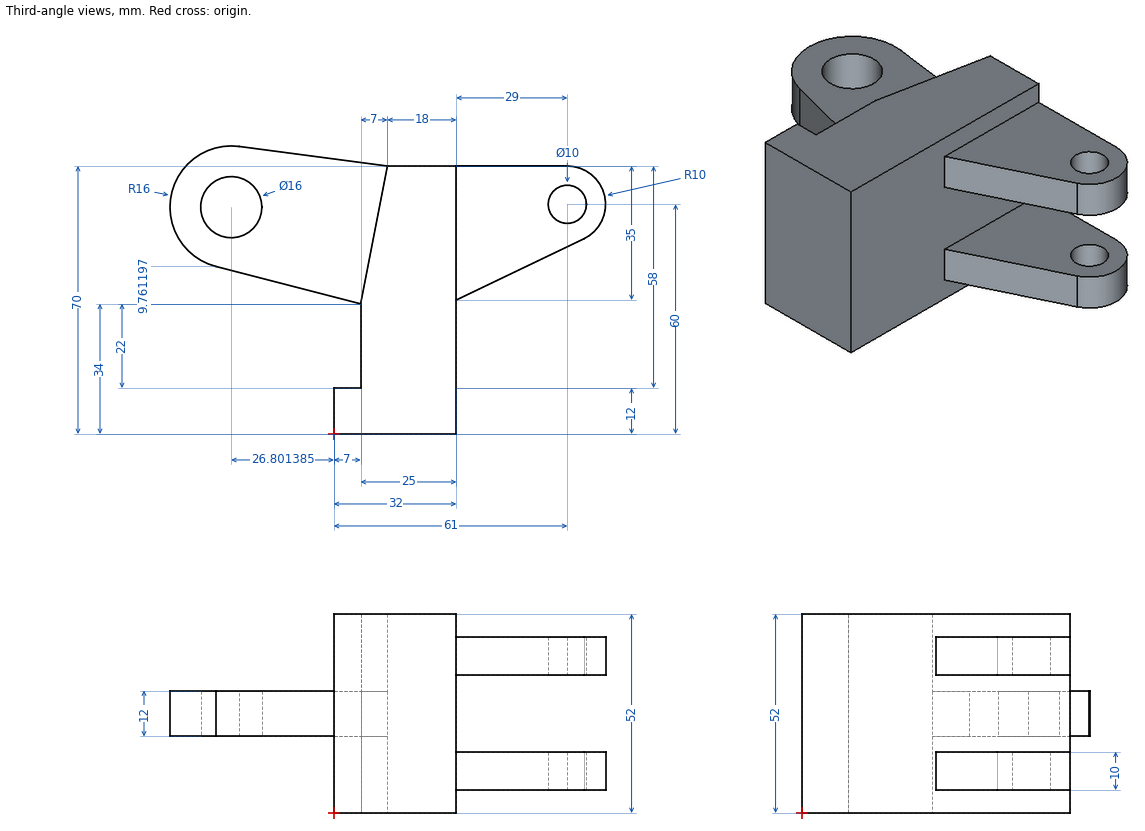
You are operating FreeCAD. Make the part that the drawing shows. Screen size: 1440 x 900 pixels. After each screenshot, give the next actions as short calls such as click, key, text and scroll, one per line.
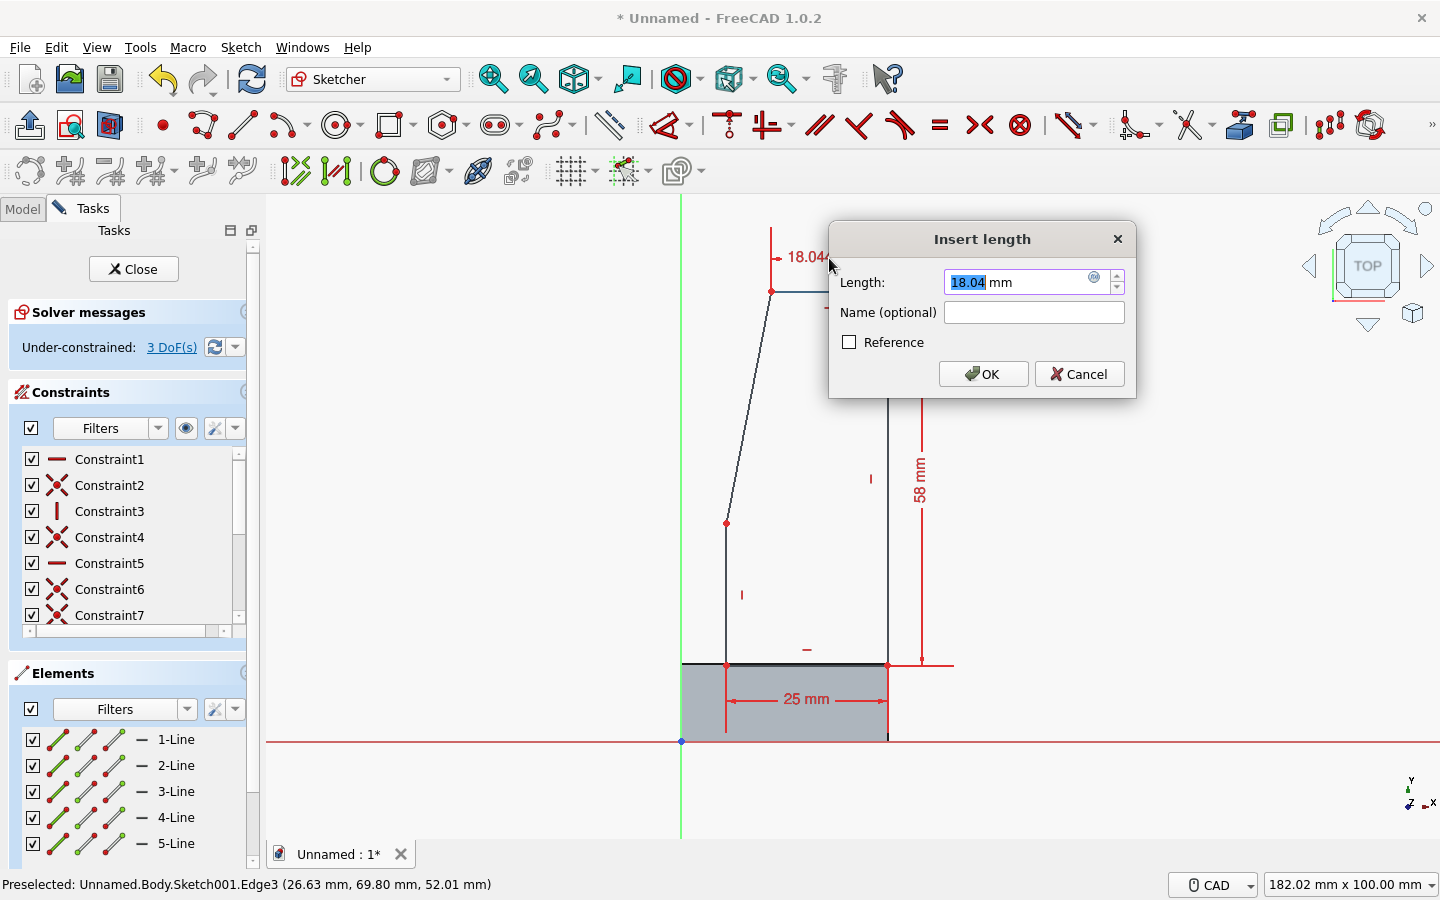
text(18)
key(Return)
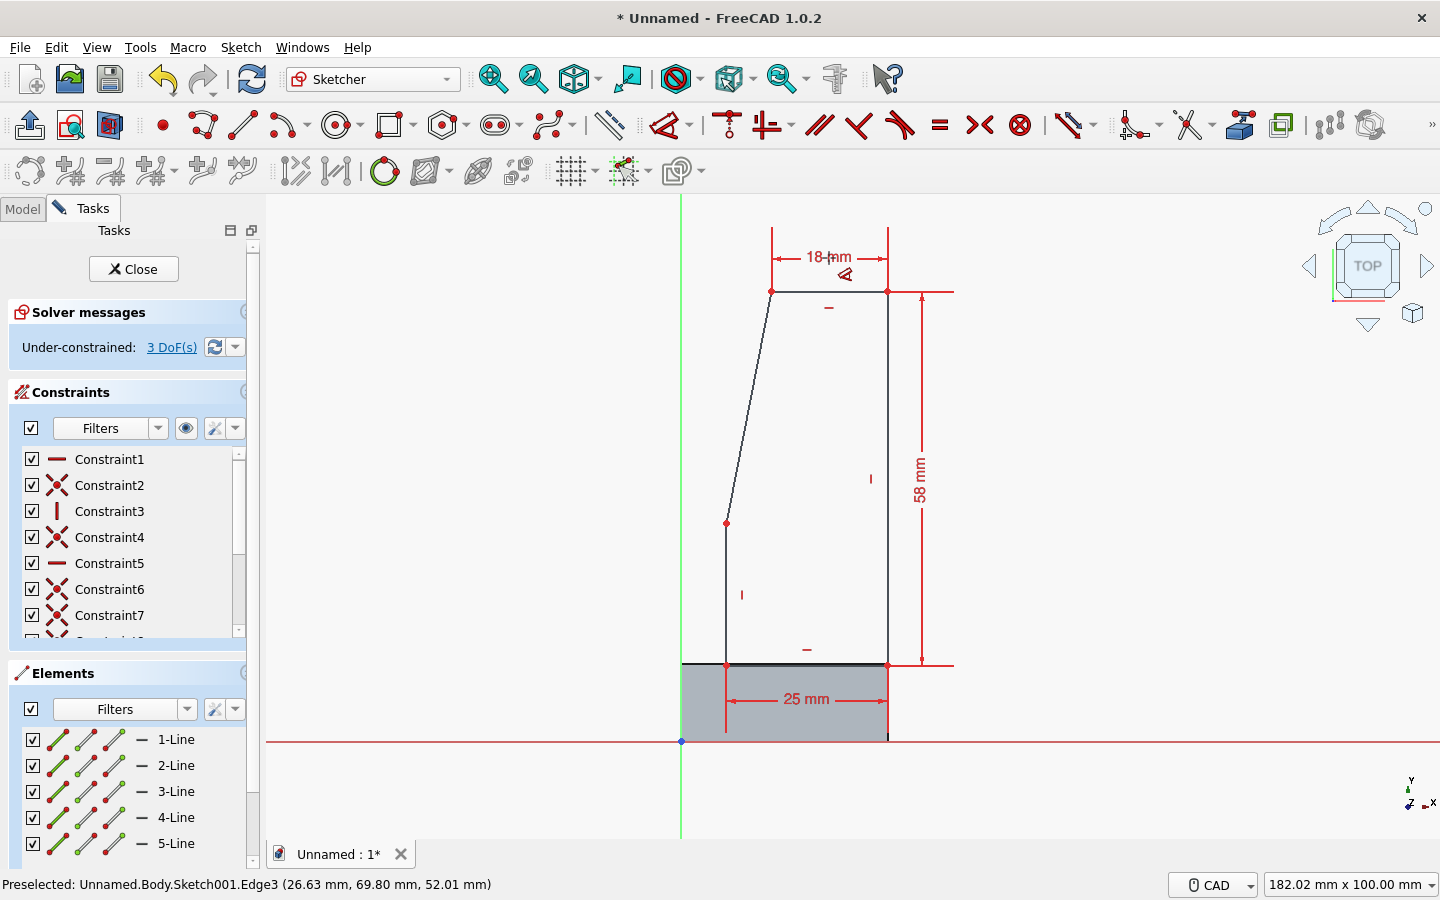
click(726, 567)
click(760, 595)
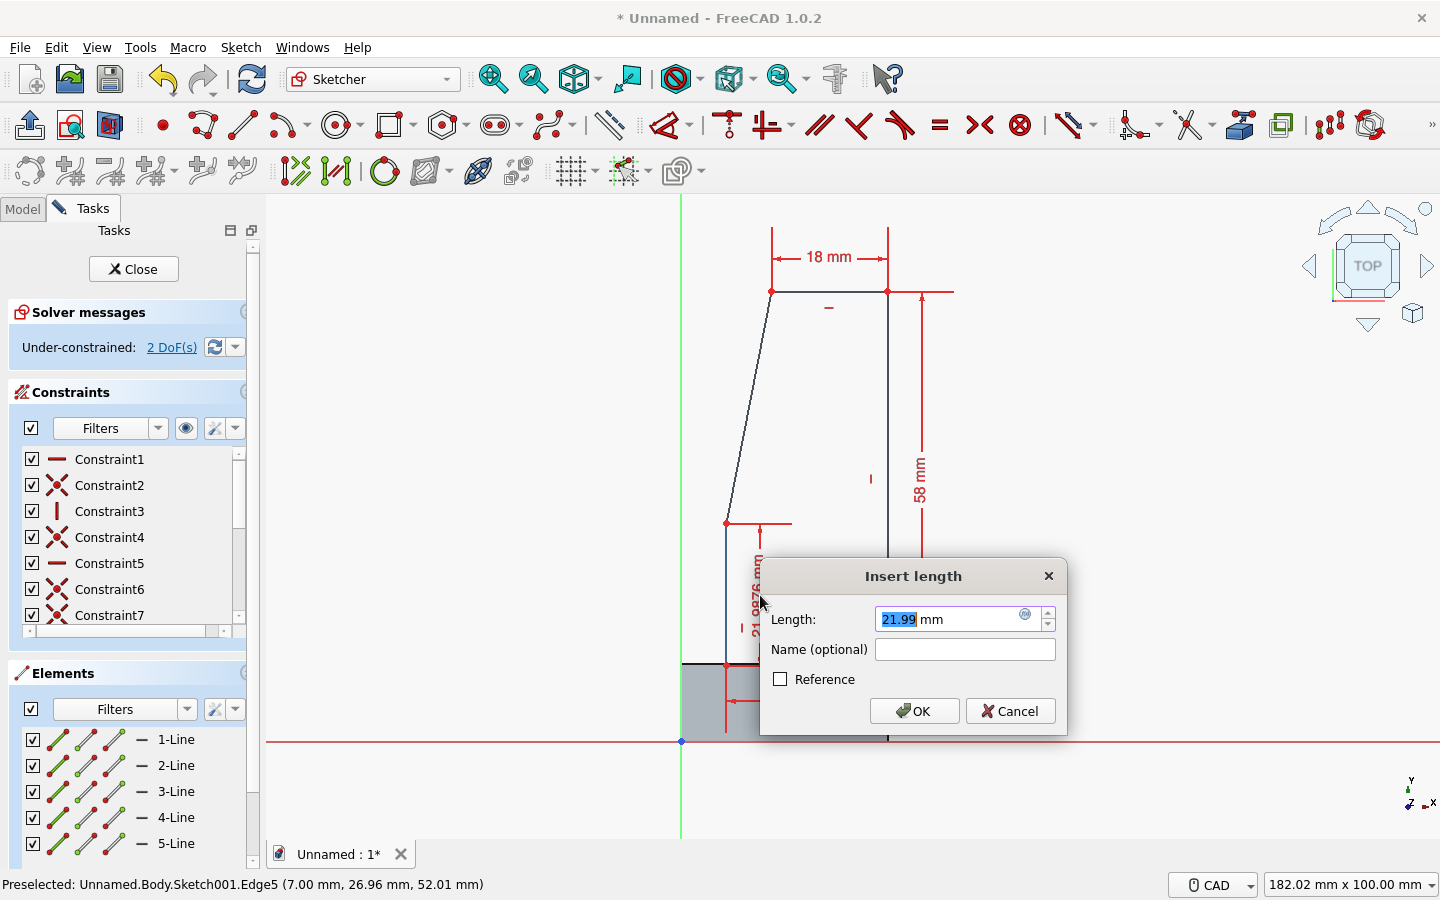
text(22)
key(Return)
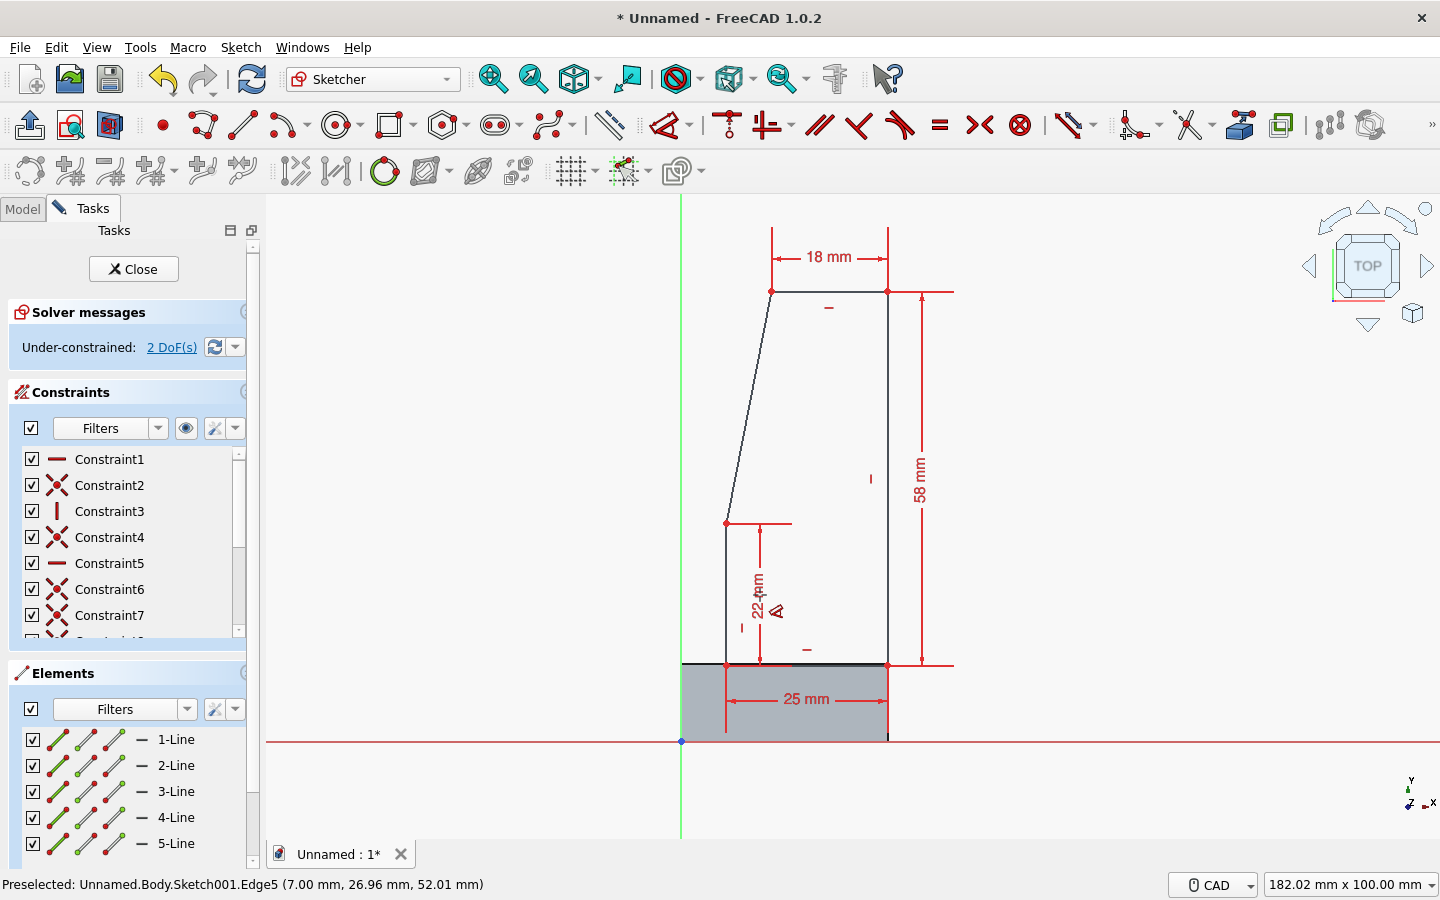
click(726, 666)
click(704, 776)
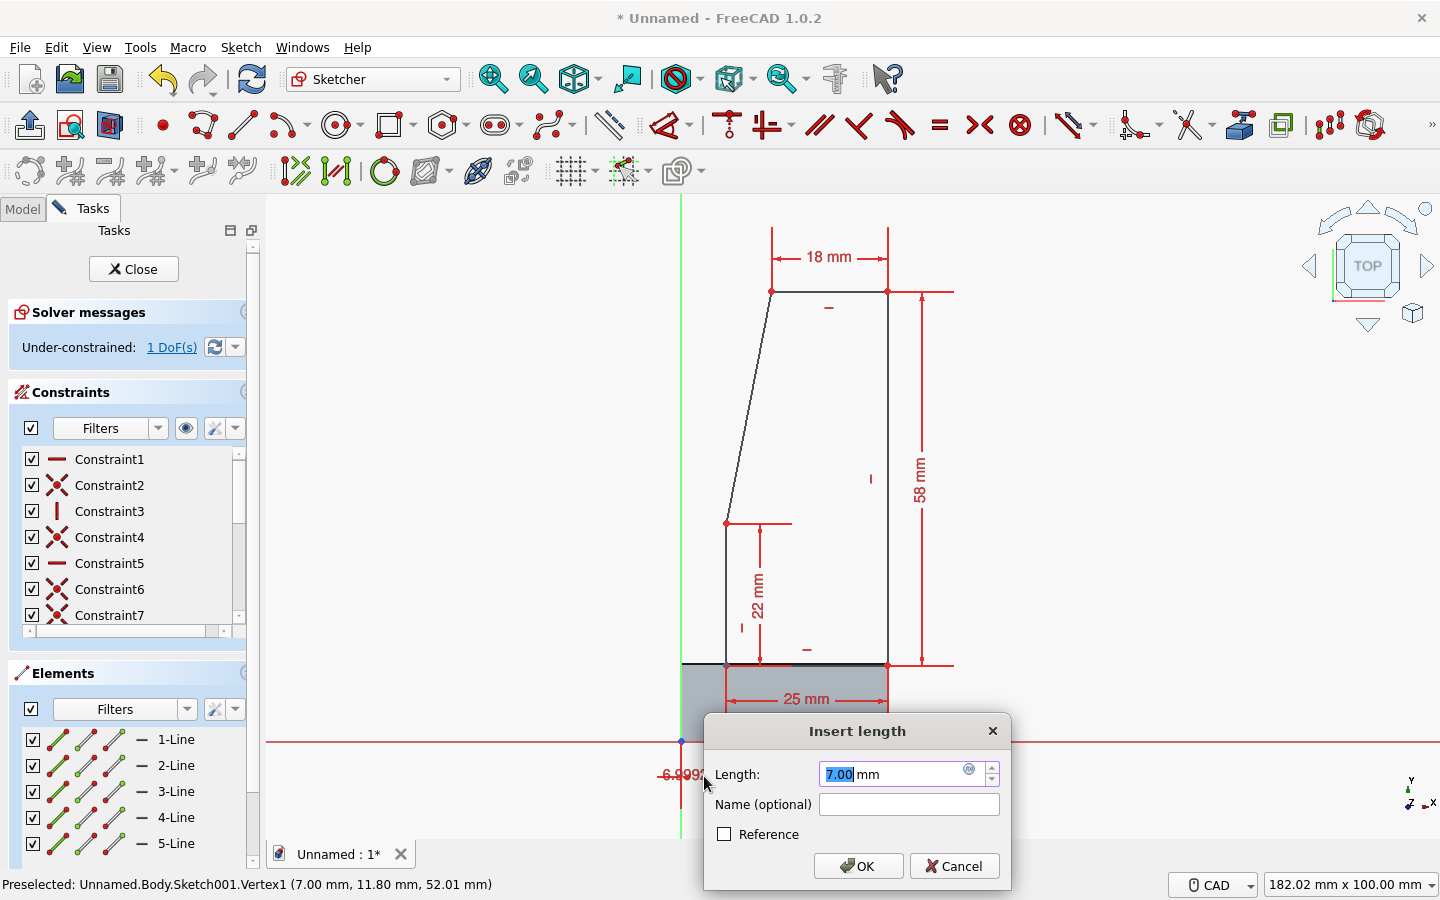
text(7)
key(Return)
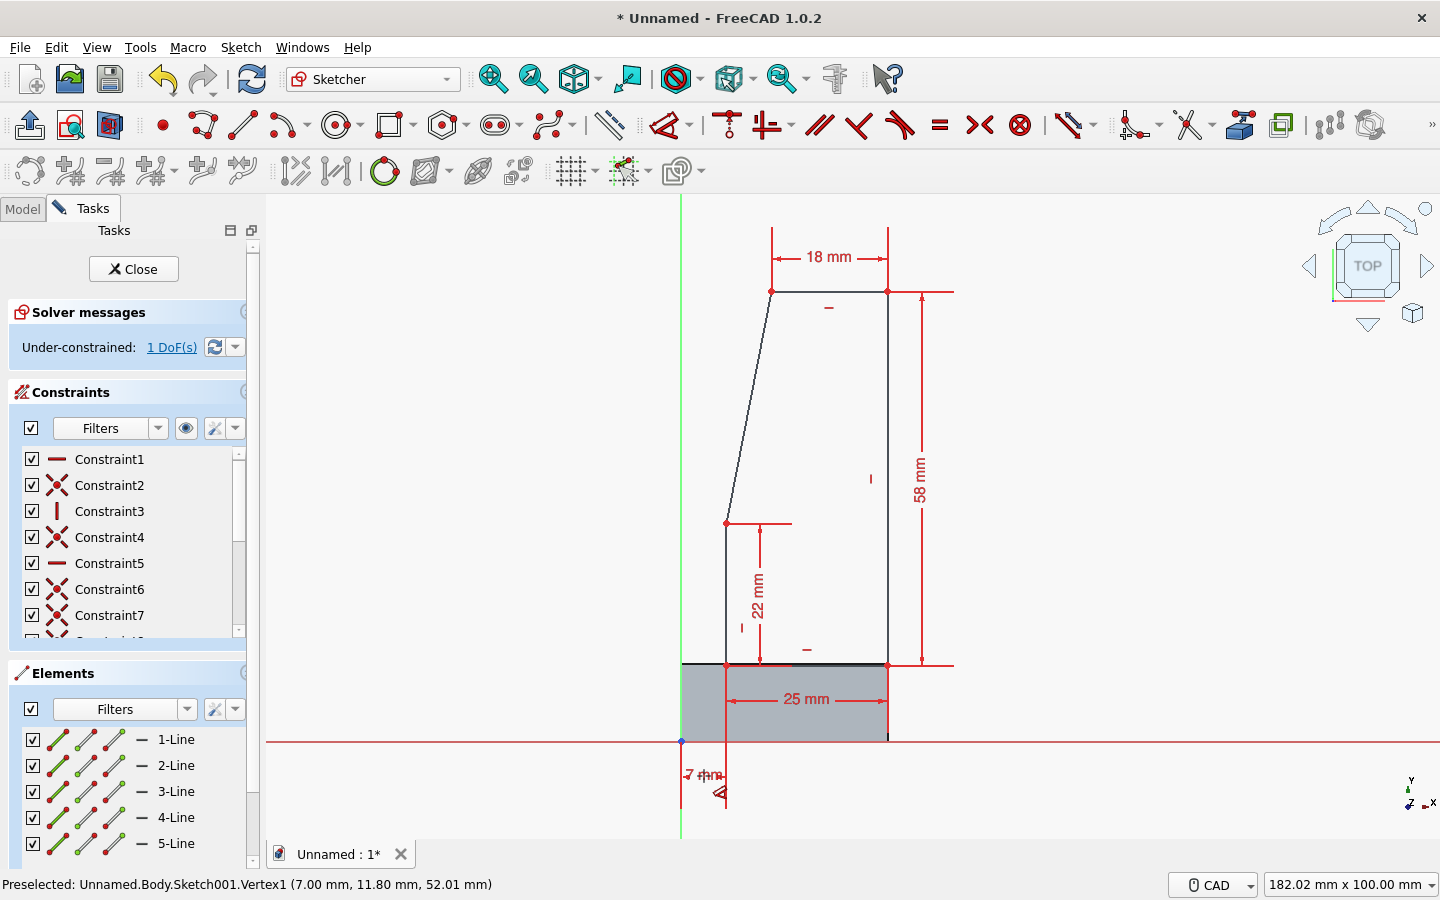
click(726, 666)
click(647, 704)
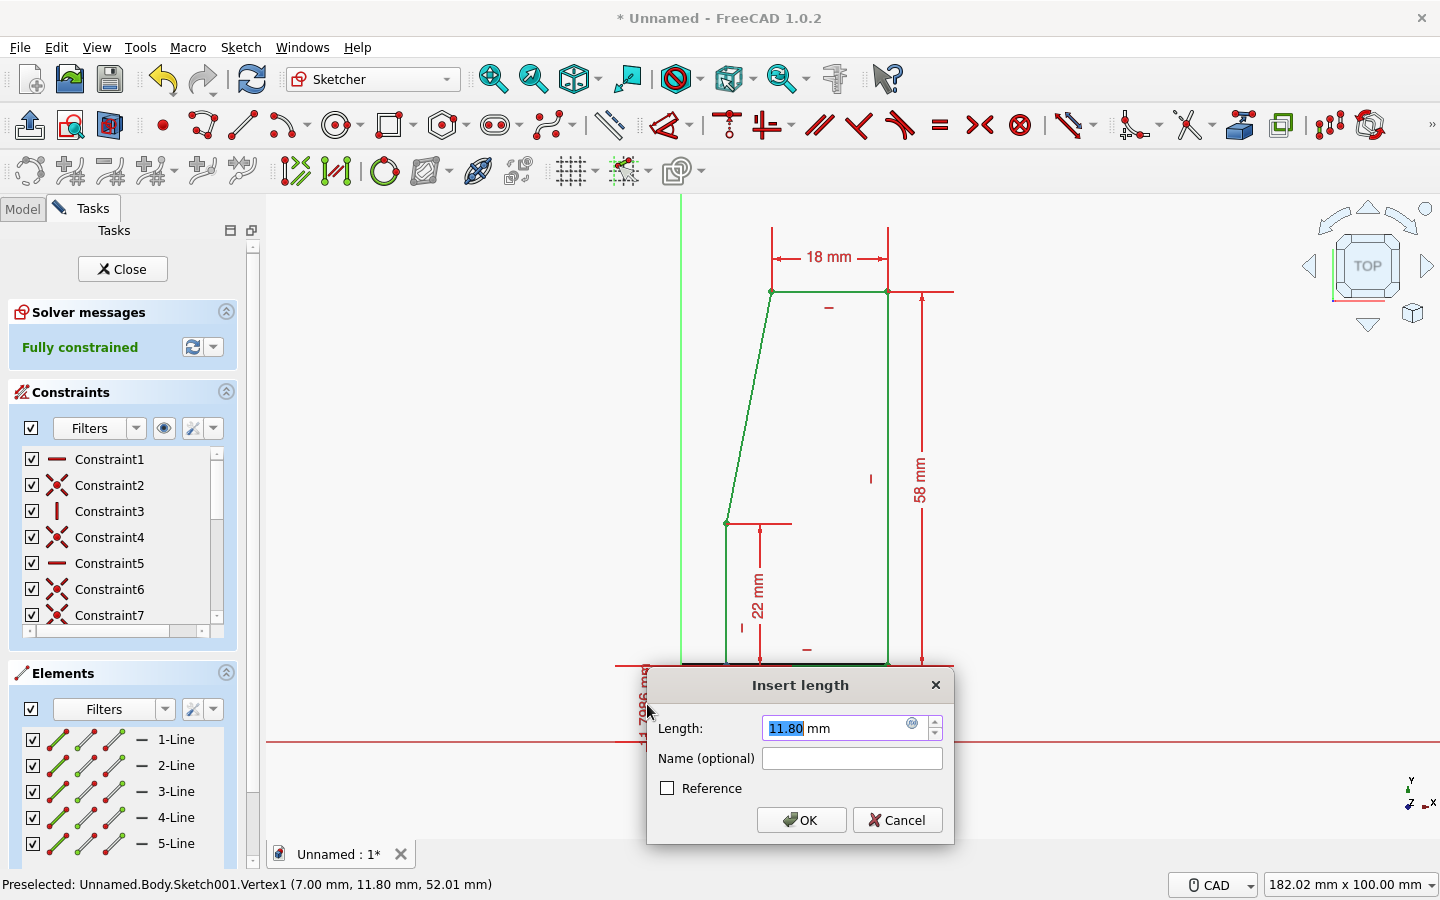
text(12)
key(Return)
key(Escape)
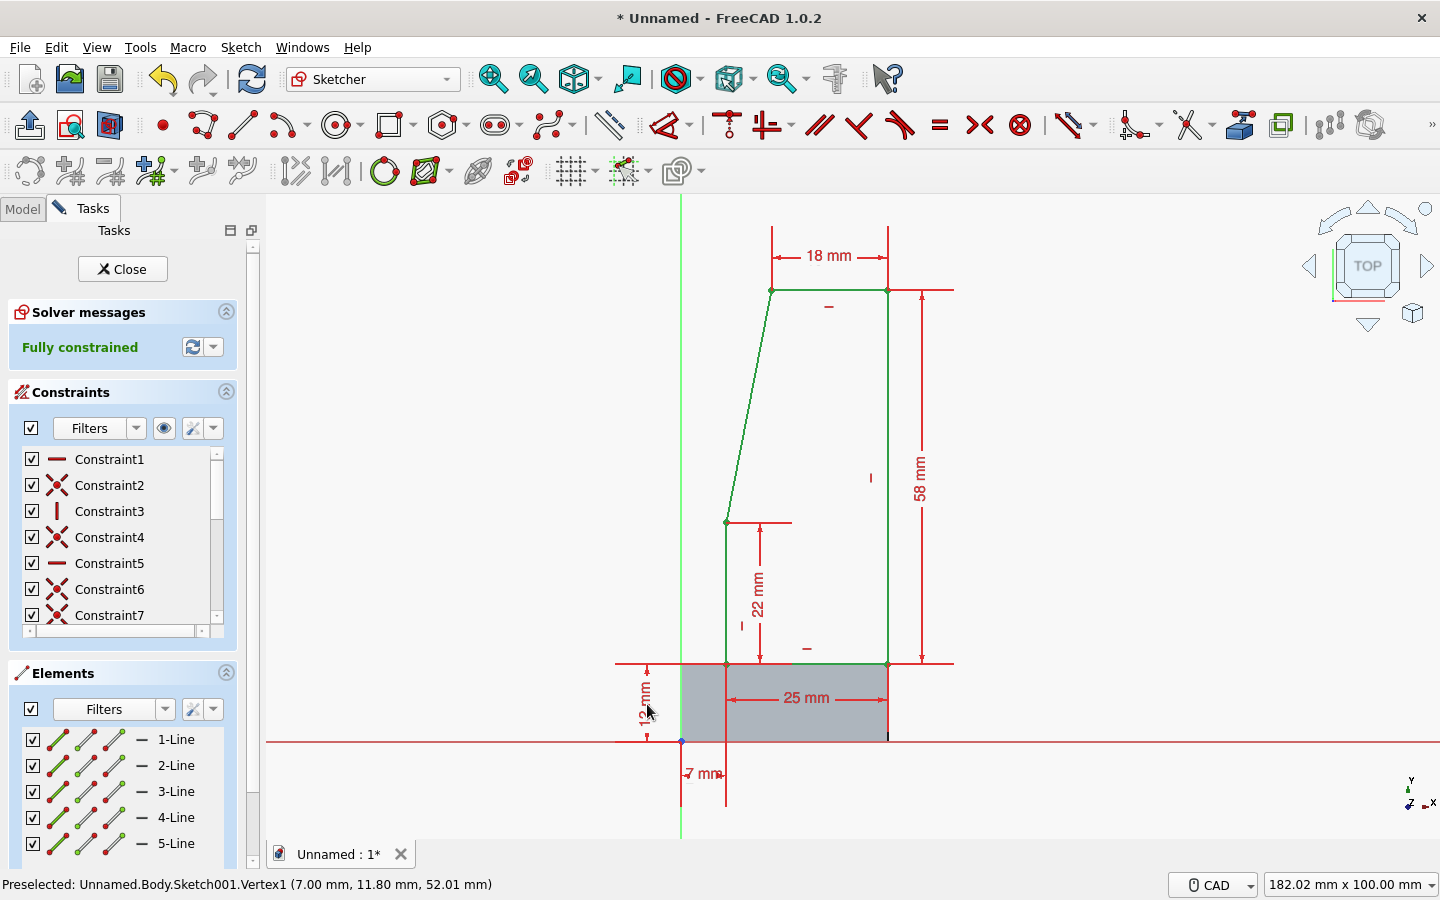
click(123, 269)